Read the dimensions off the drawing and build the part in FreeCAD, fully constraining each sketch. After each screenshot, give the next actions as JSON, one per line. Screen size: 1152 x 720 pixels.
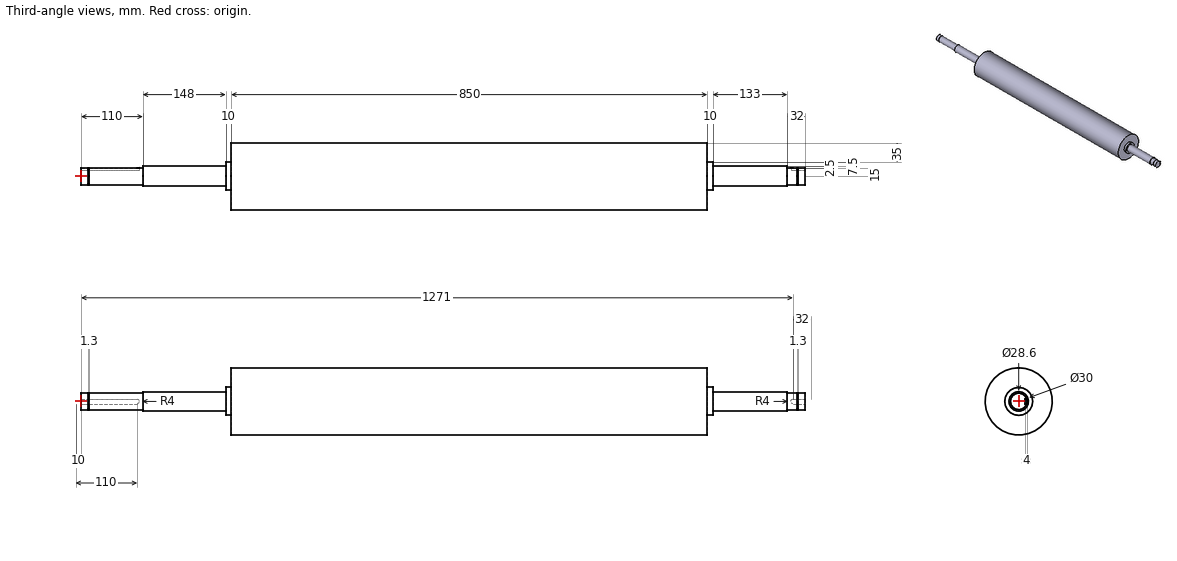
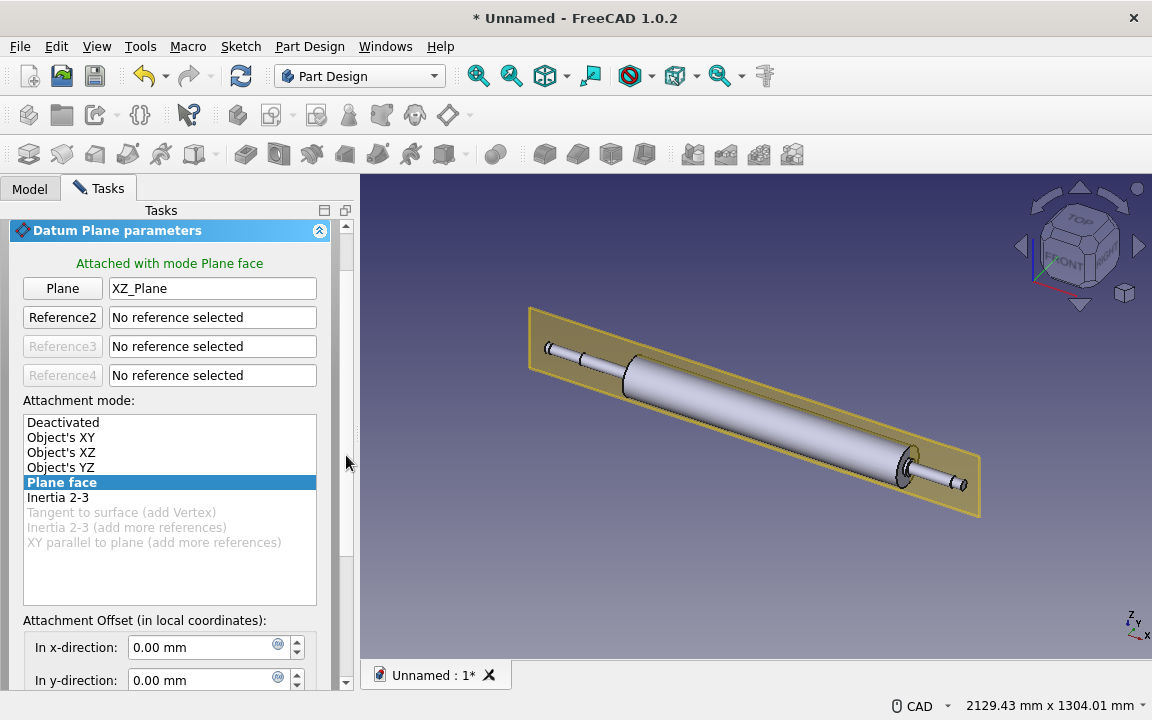
{"action": "left_click", "coordinate": [127, 249]}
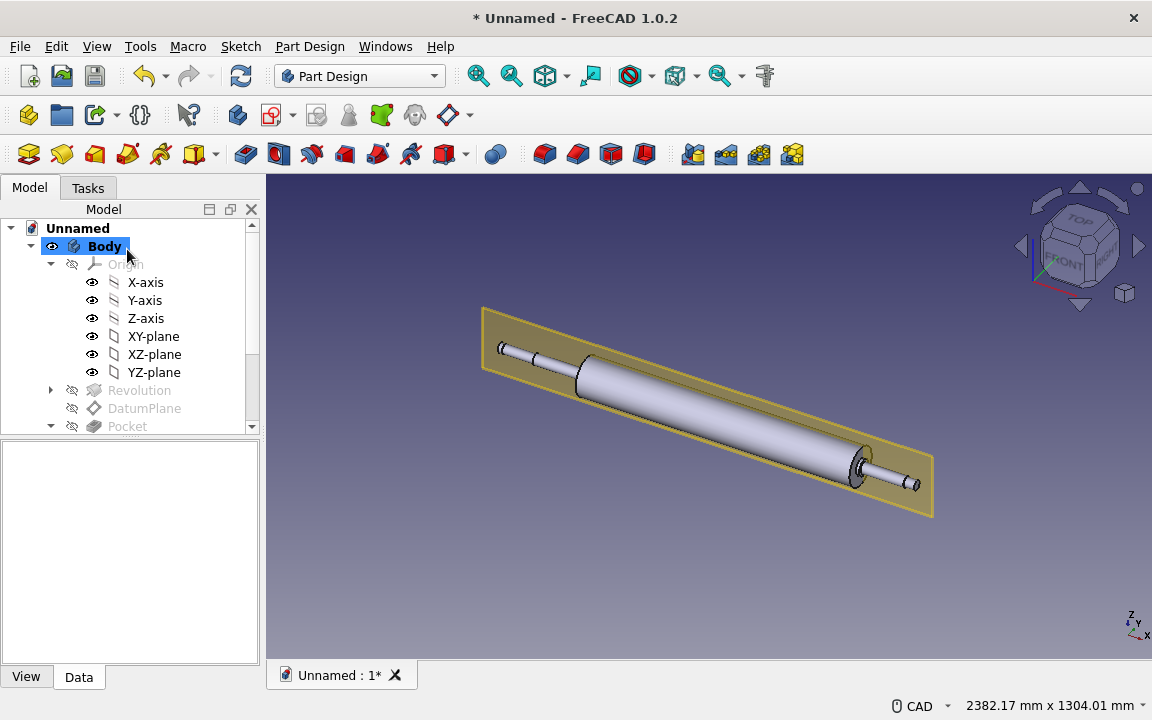
{"action": "scroll", "coordinate": [101, 332], "scroll_direction": "down", "scroll_amount": 3}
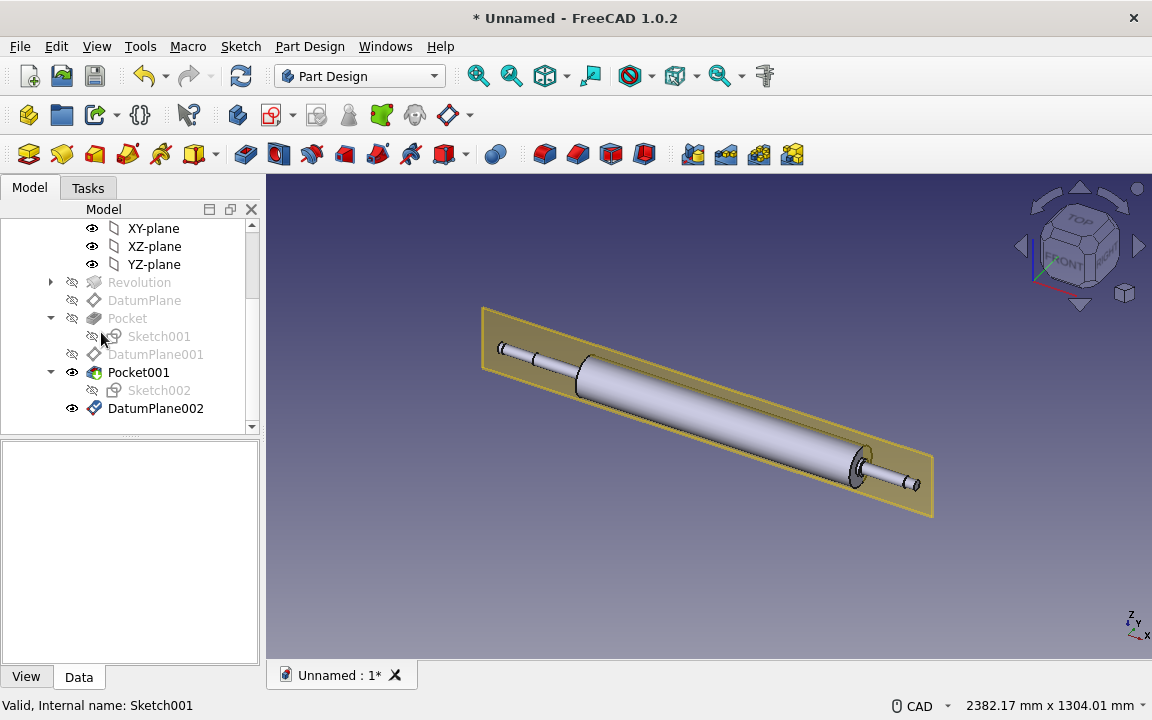
{"action": "left_click", "coordinate": [117, 408]}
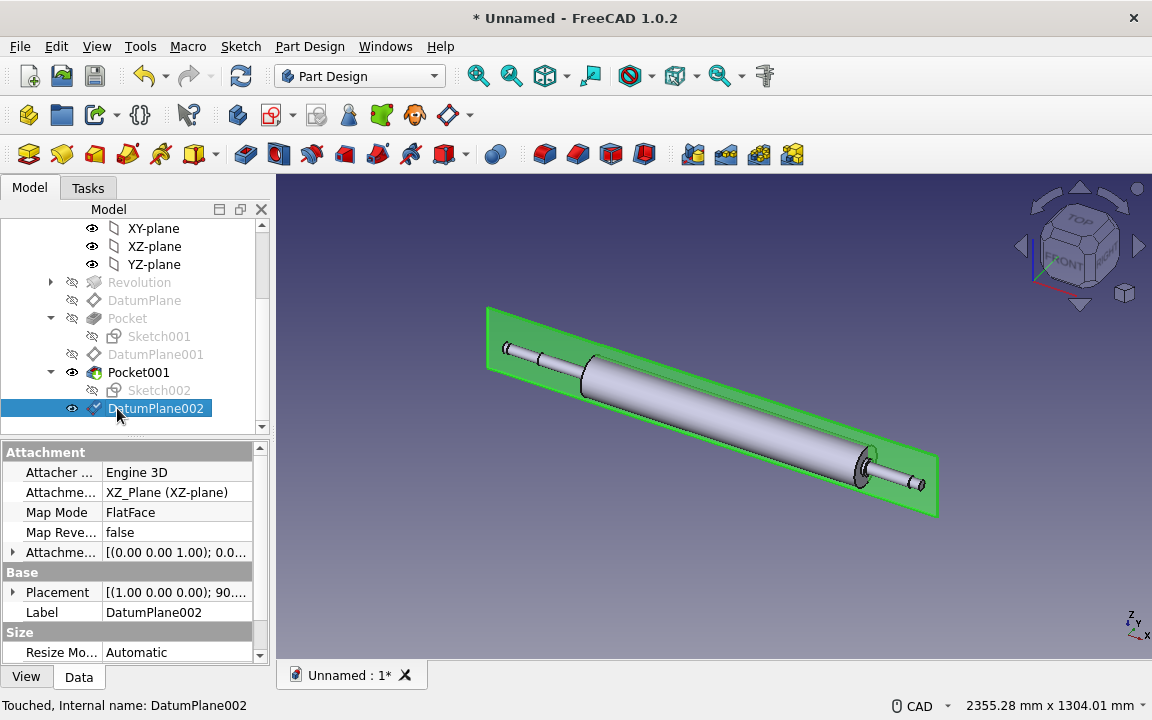
{"action": "left_click", "coordinate": [270, 116]}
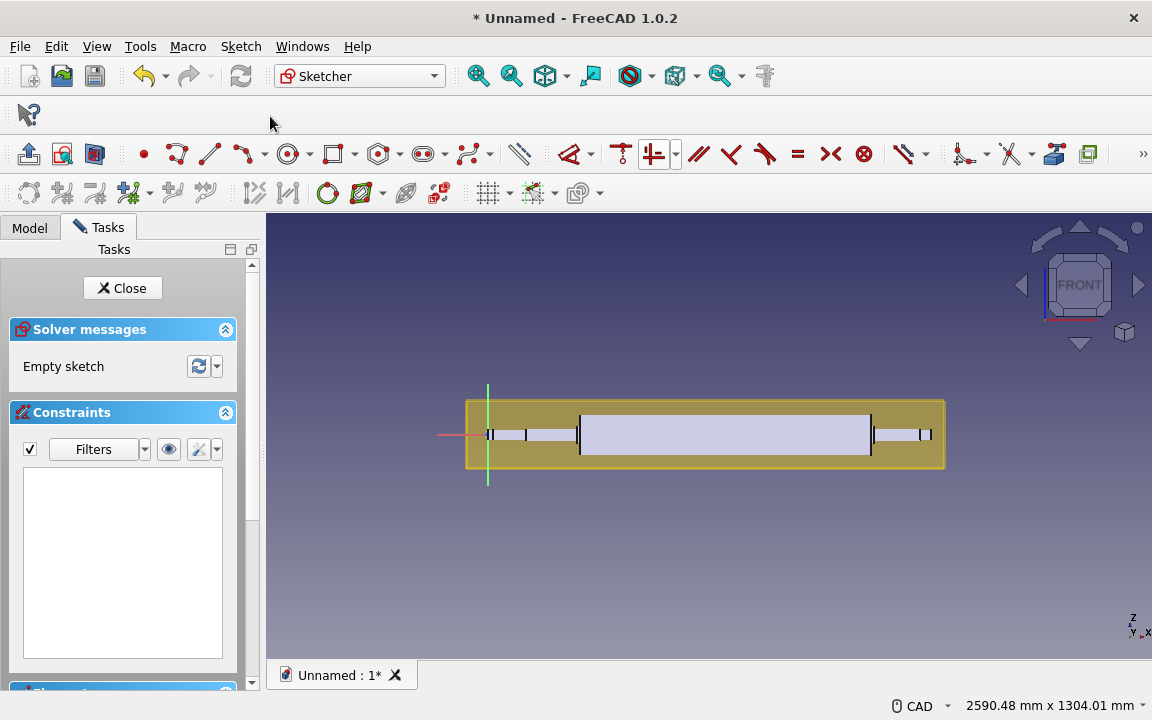
{"action": "left_click", "coordinate": [95, 154]}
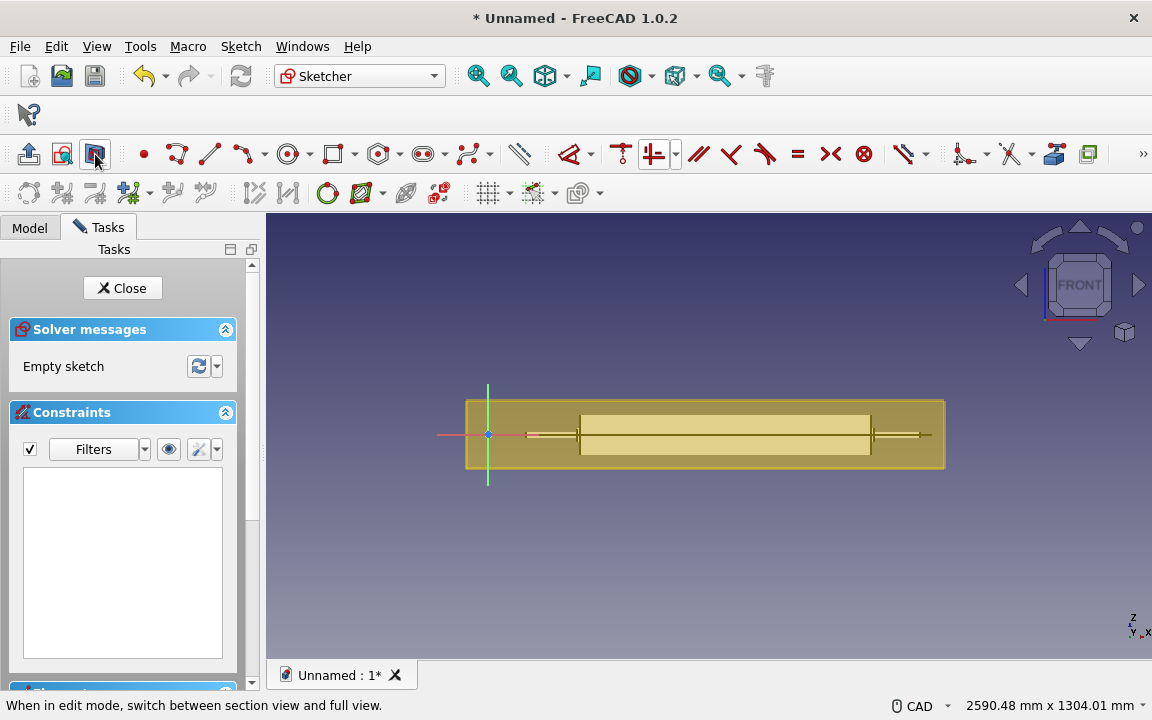
{"action": "scroll", "coordinate": [943, 435], "scroll_direction": "up", "scroll_amount": 15}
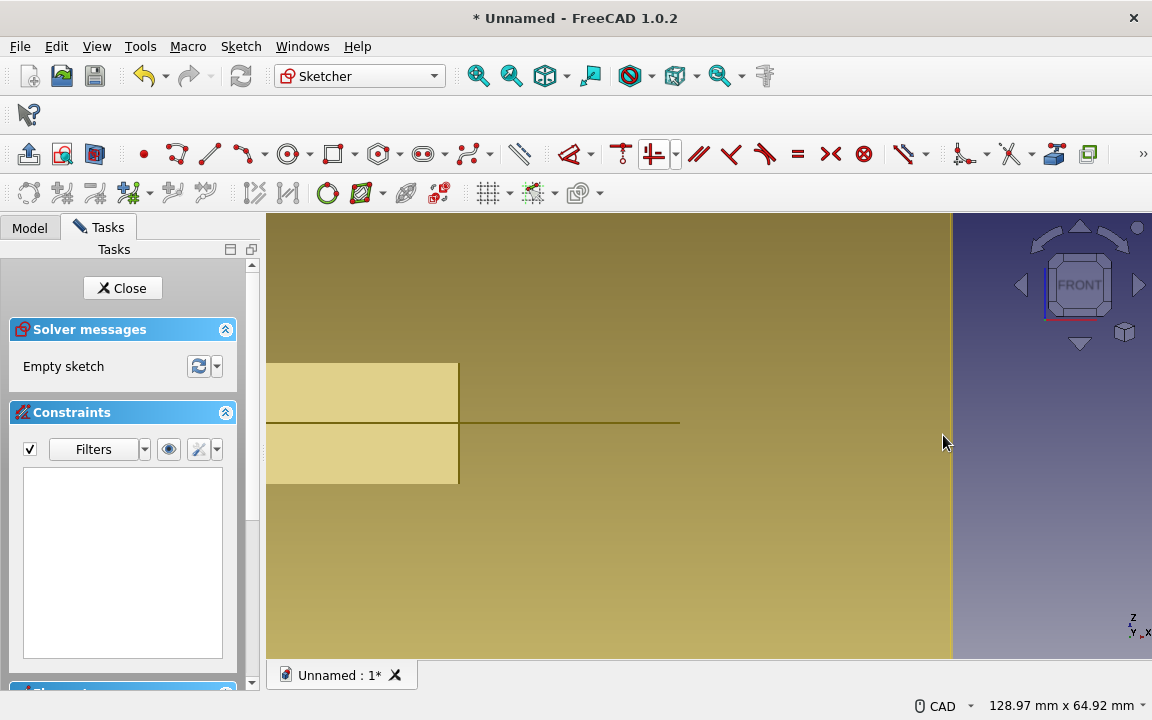
{"action": "scroll", "coordinate": [604, 408], "scroll_direction": "up", "scroll_amount": 3}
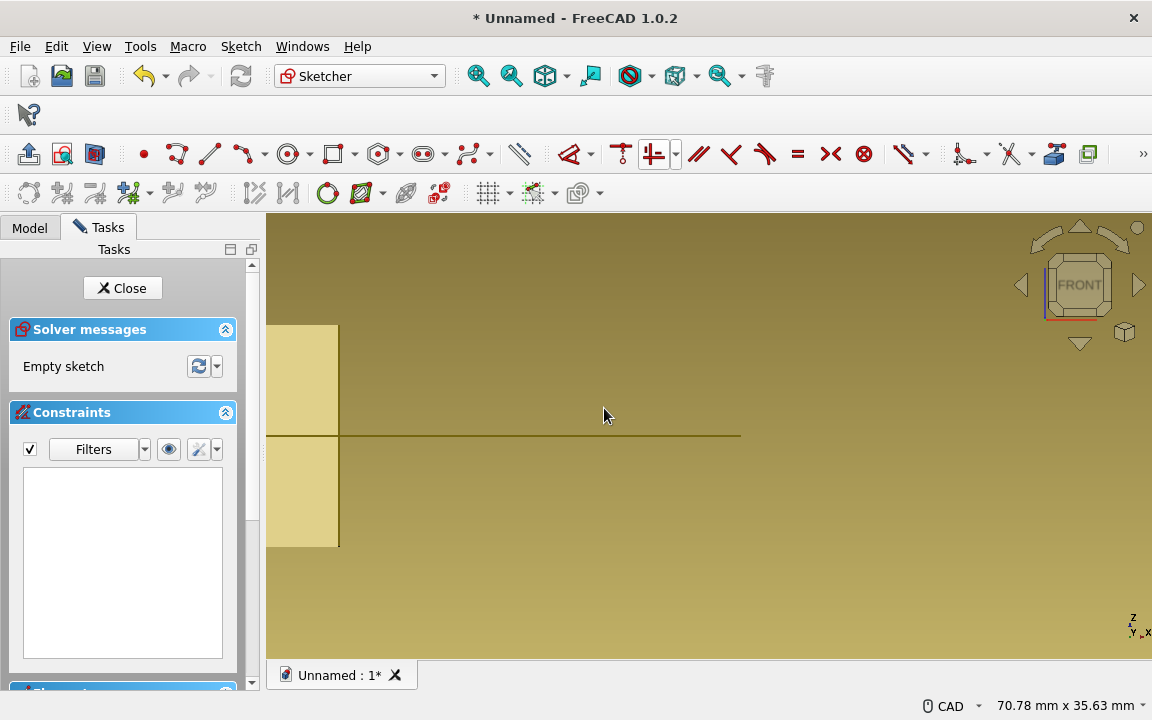
{"action": "key", "text": "g m"}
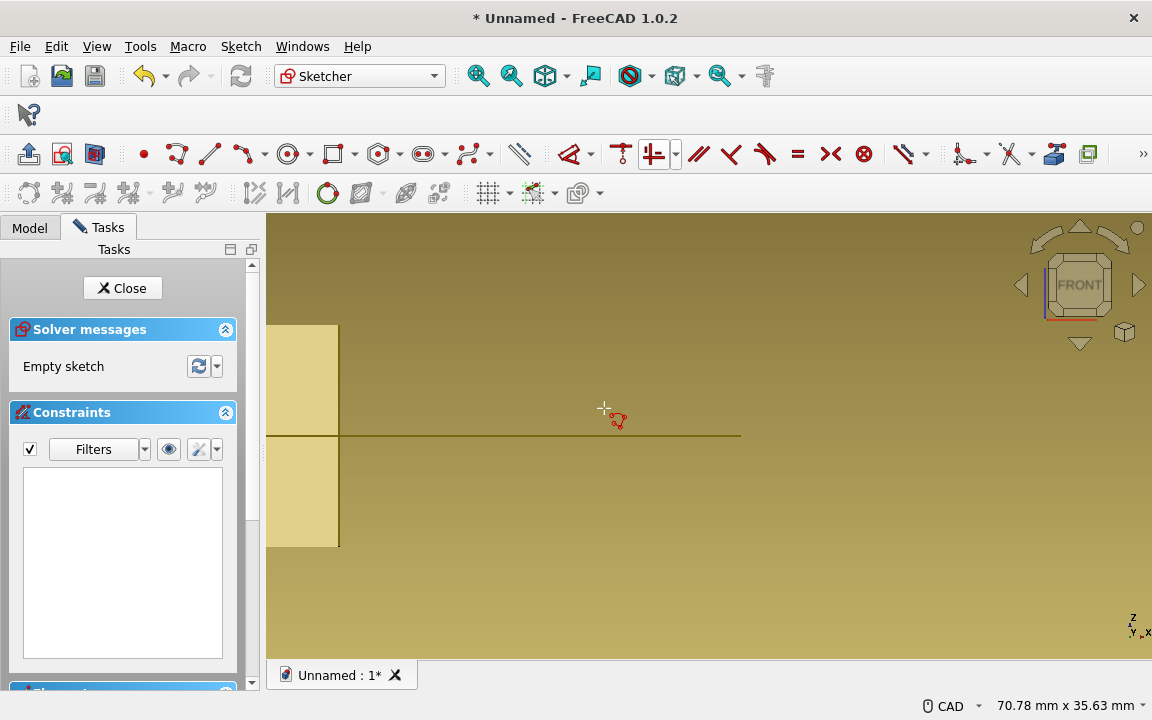
{"action": "left_click", "coordinate": [465, 386]}
{"action": "left_click", "coordinate": [865, 386]}
{"action": "left_click", "coordinate": [865, 486]}
{"action": "left_click", "coordinate": [465, 486]}
{"action": "right_click", "coordinate": [465, 486]}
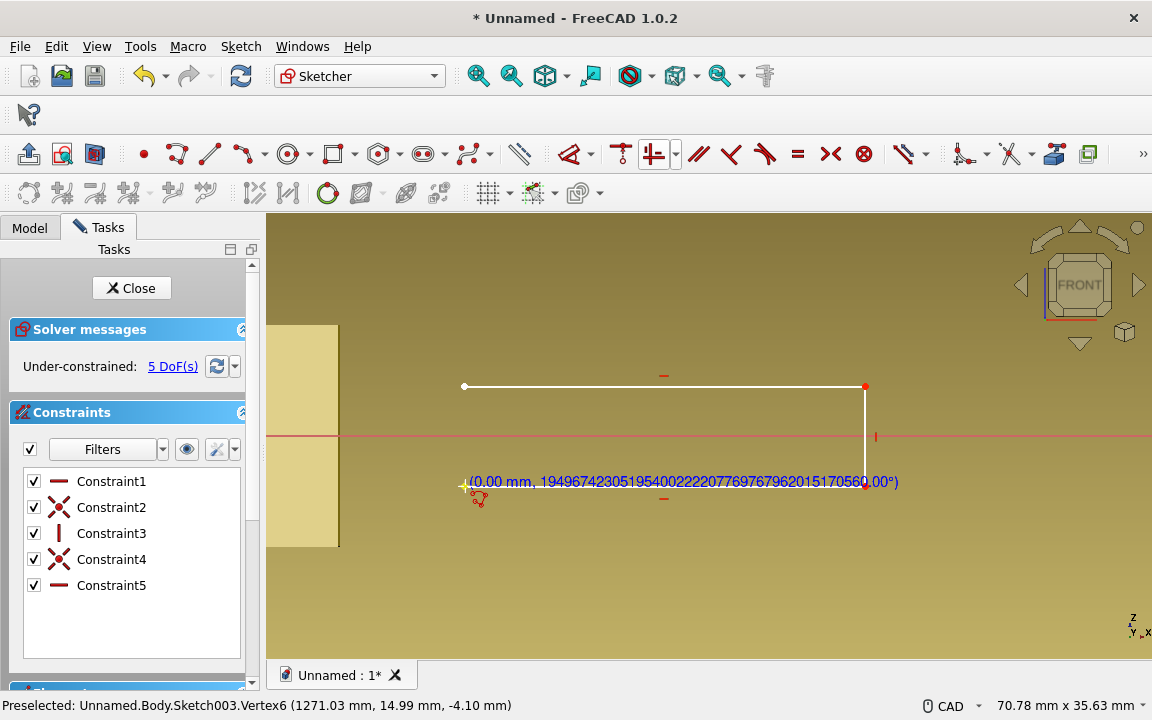
{"action": "key", "text": "g 3 a"}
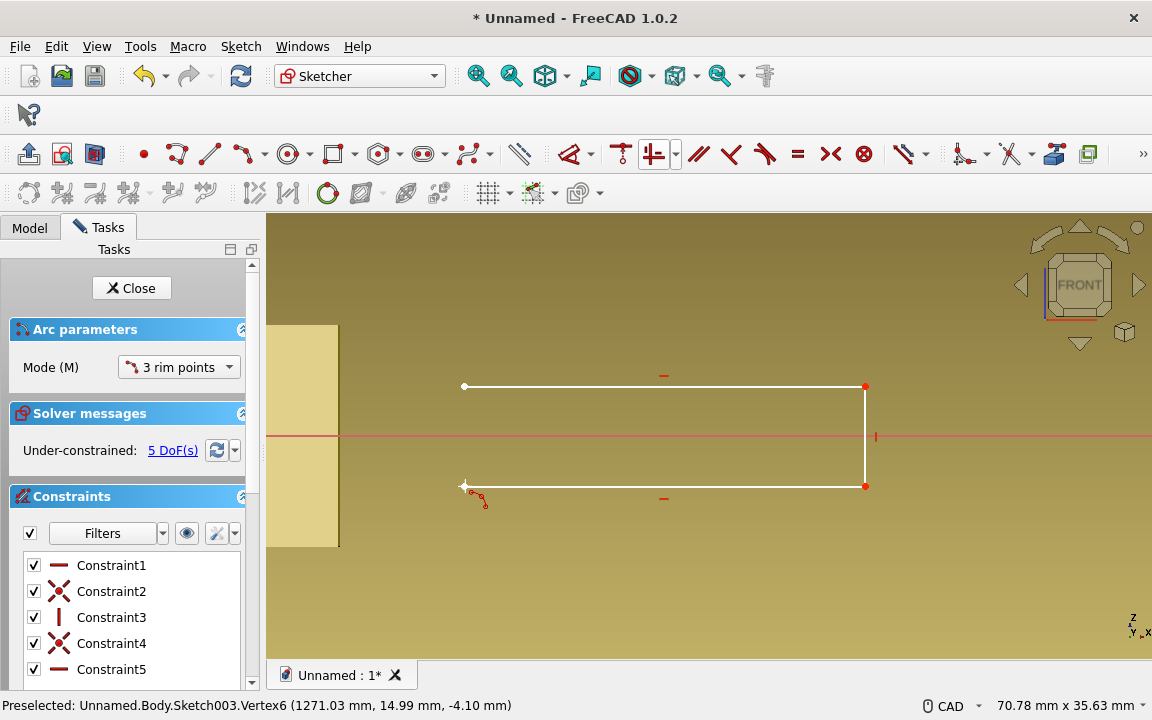
{"action": "left_click", "coordinate": [465, 487]}
{"action": "left_click", "coordinate": [465, 387]}
{"action": "left_click", "coordinate": [417, 420]}
{"action": "key", "text": "Escape"}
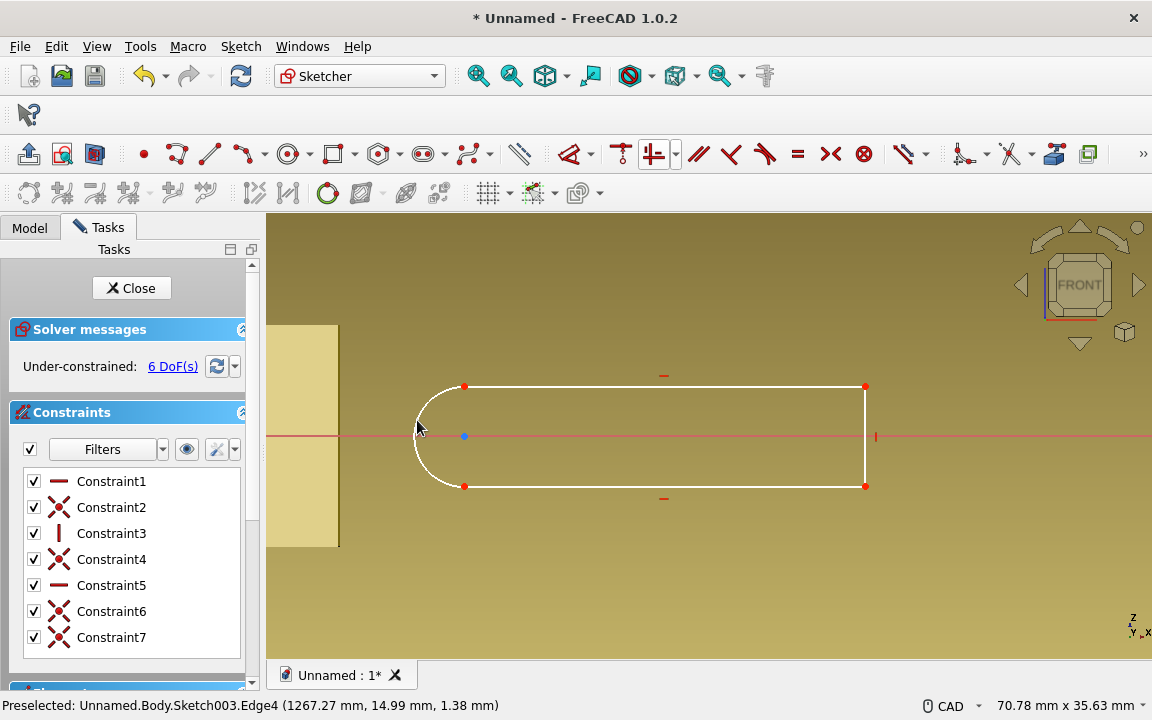
{"action": "left_click", "coordinate": [585, 387]}